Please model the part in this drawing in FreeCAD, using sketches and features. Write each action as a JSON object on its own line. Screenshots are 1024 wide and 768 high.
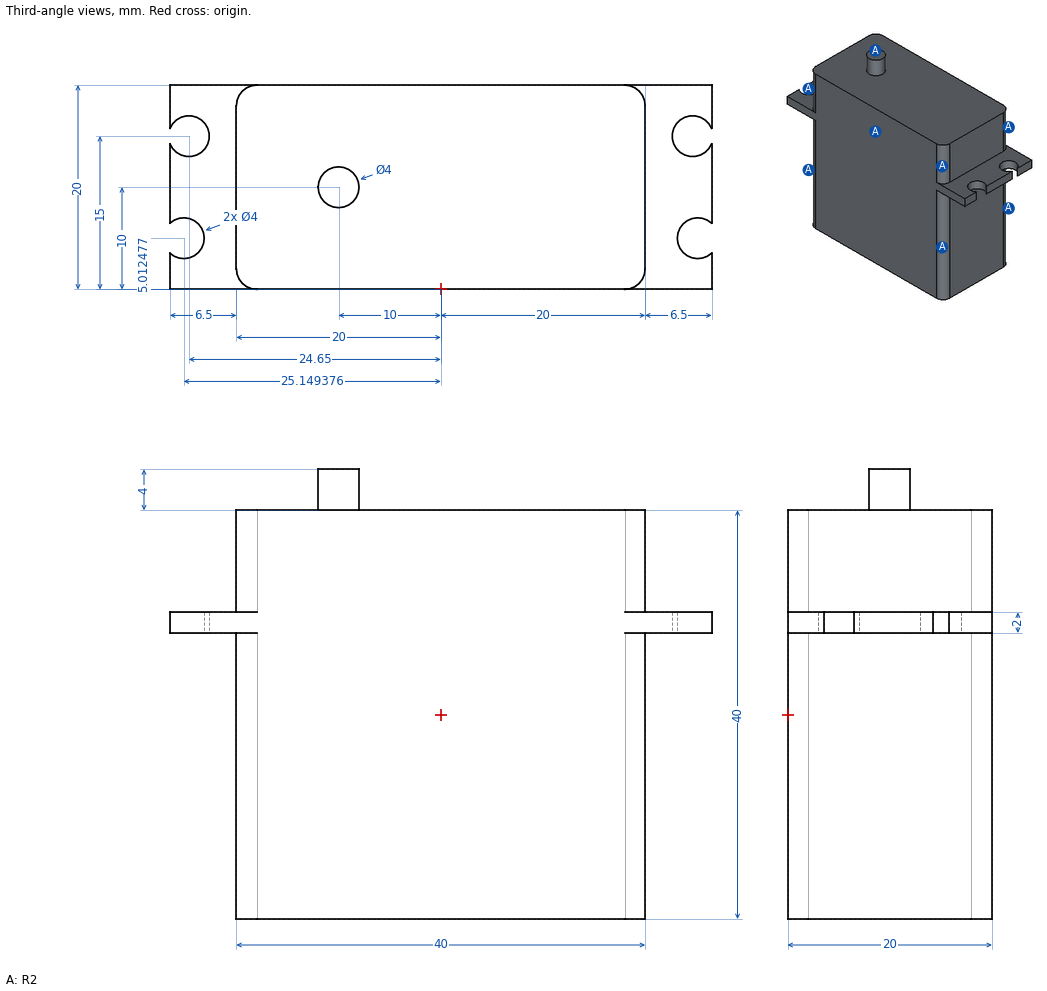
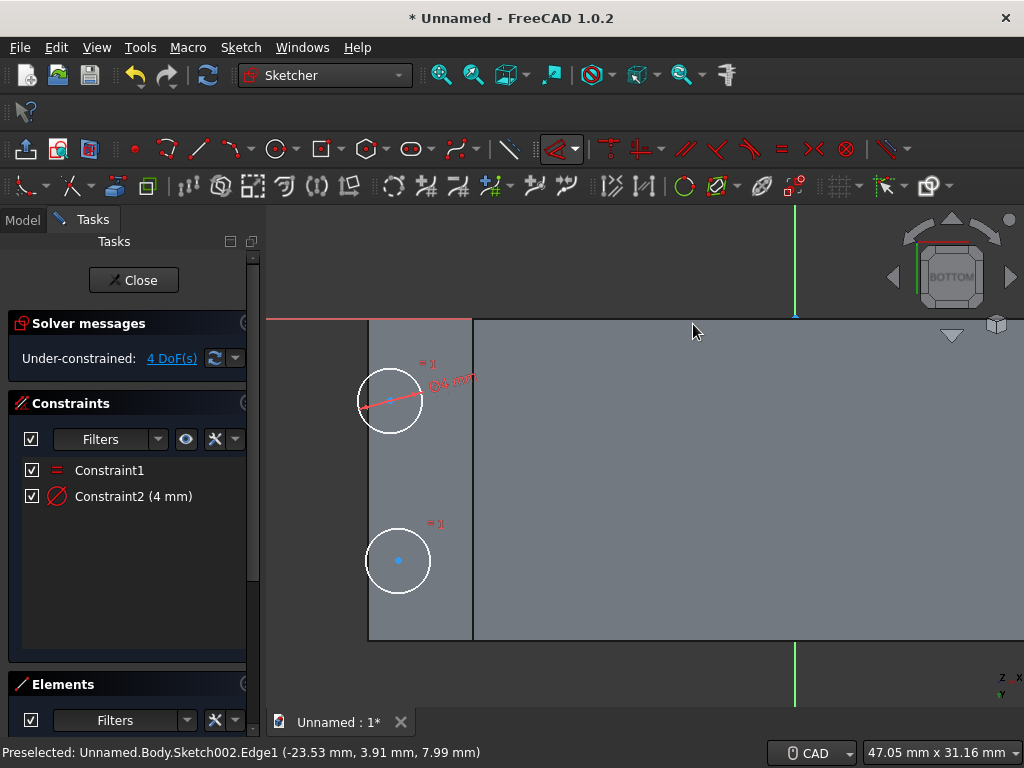
{"action": "left_click", "coordinate": [398, 561]}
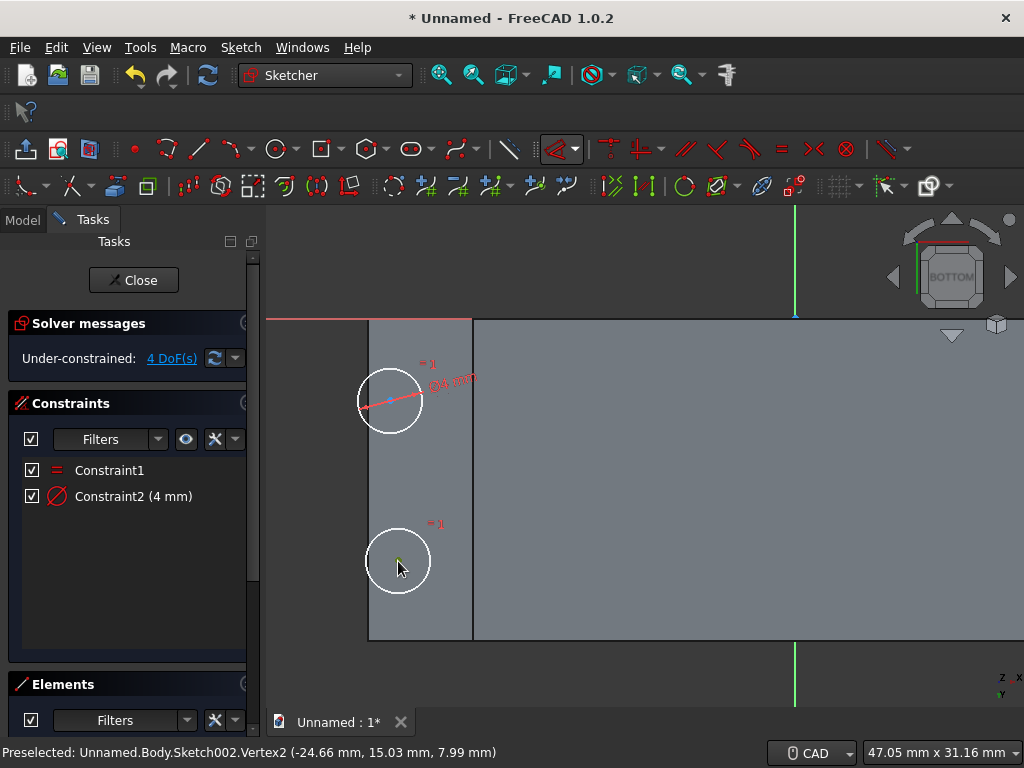
{"action": "left_click", "coordinate": [578, 150]}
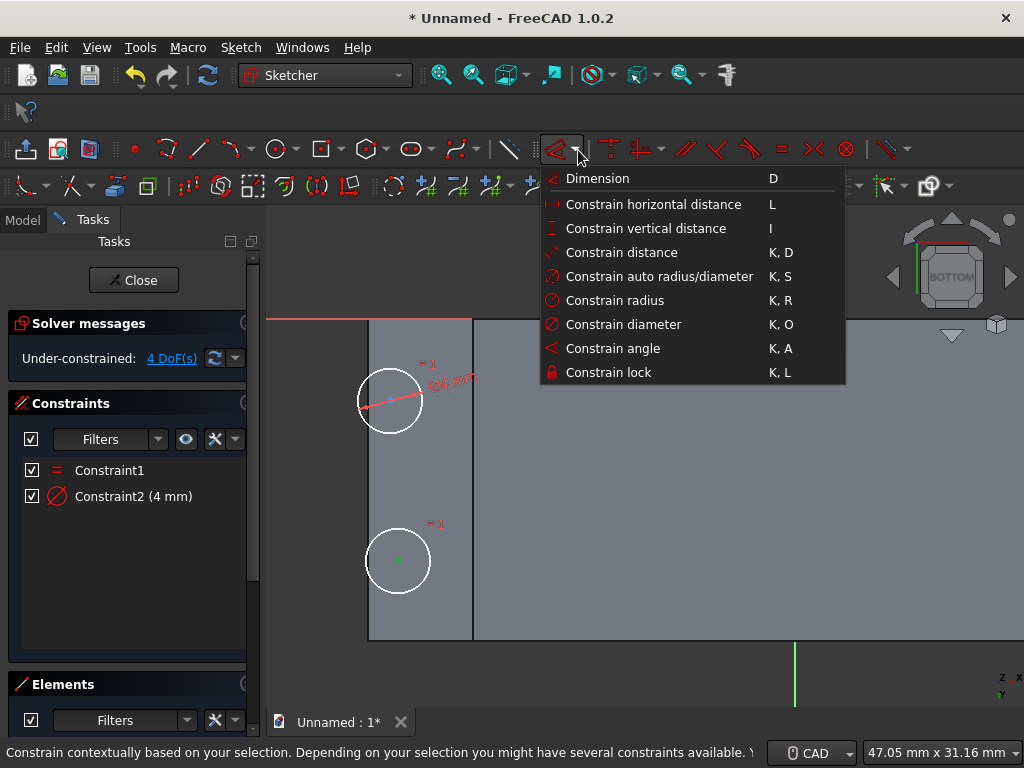
{"action": "left_click", "coordinate": [693, 228]}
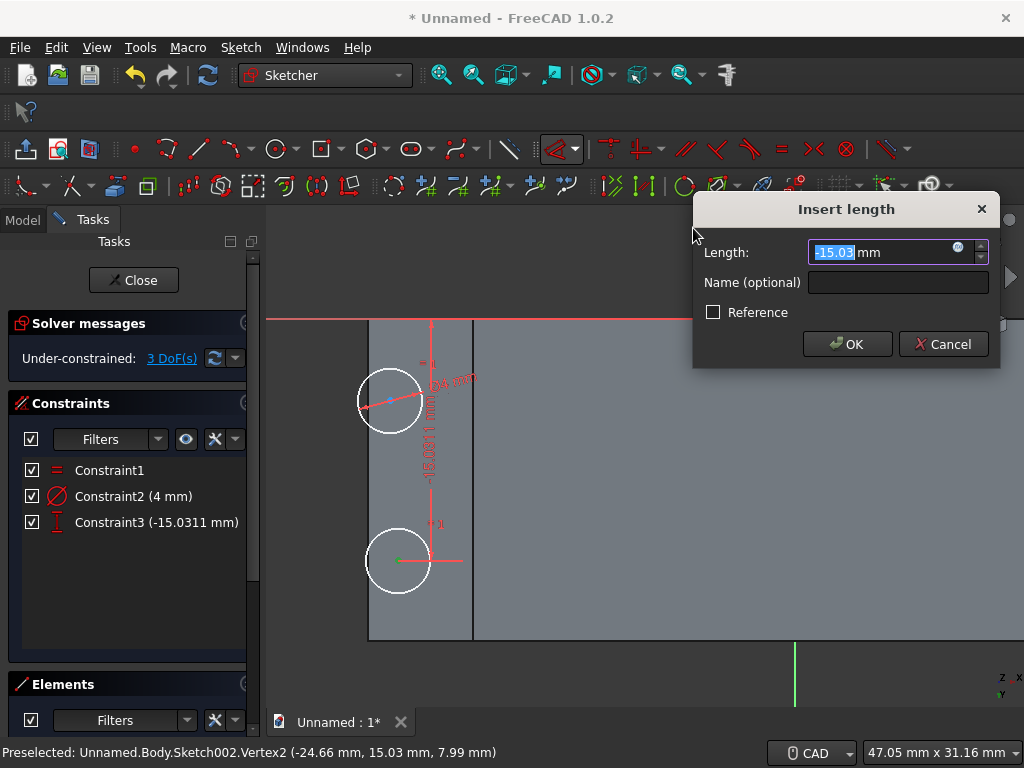
{"action": "type", "text": "-15"}
{"action": "key", "text": "Return"}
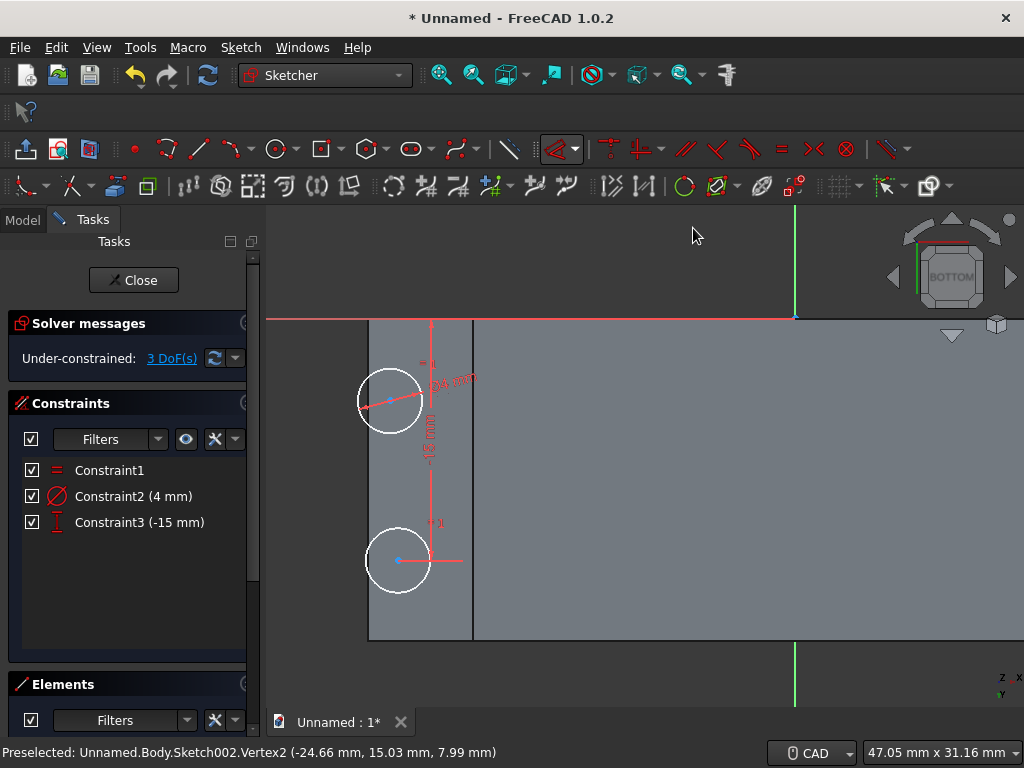
{"action": "left_click", "coordinate": [398, 560]}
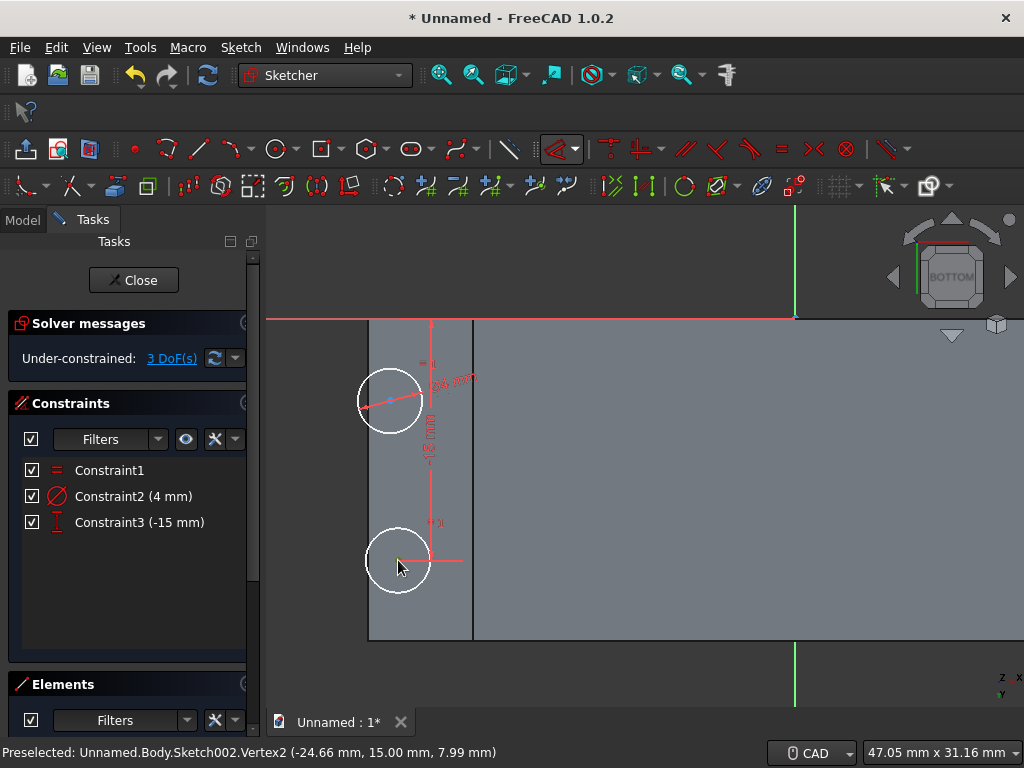
{"action": "key", "text": "l"}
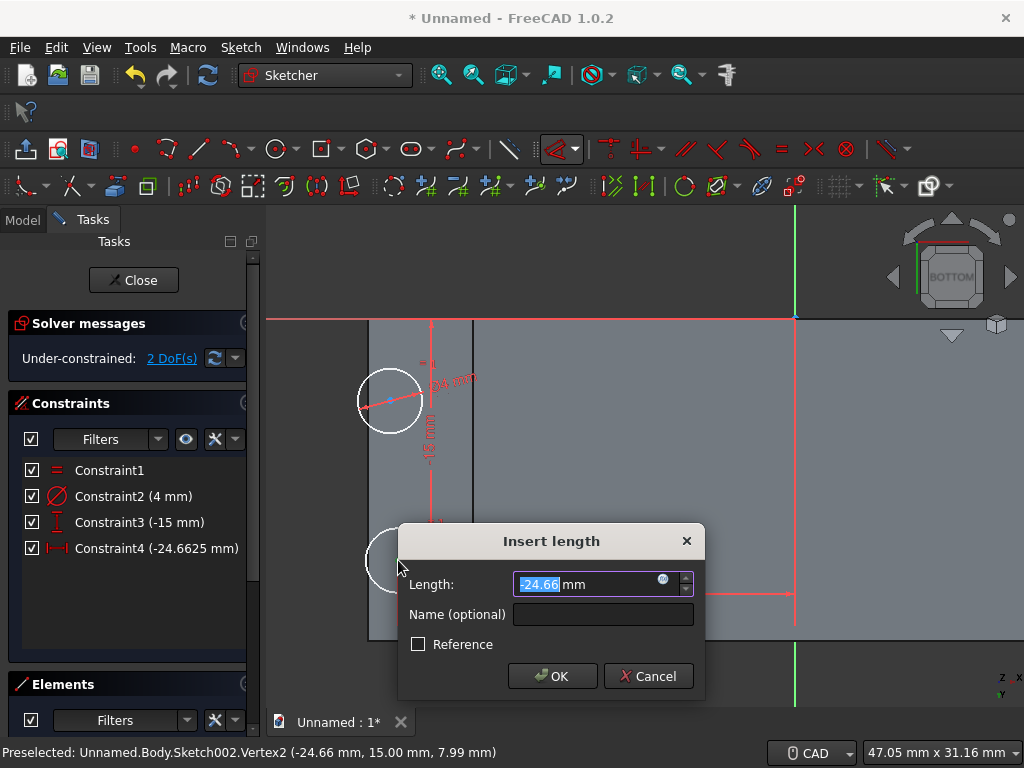
{"action": "type", "text": "-24.65"}
{"action": "key", "text": "Return"}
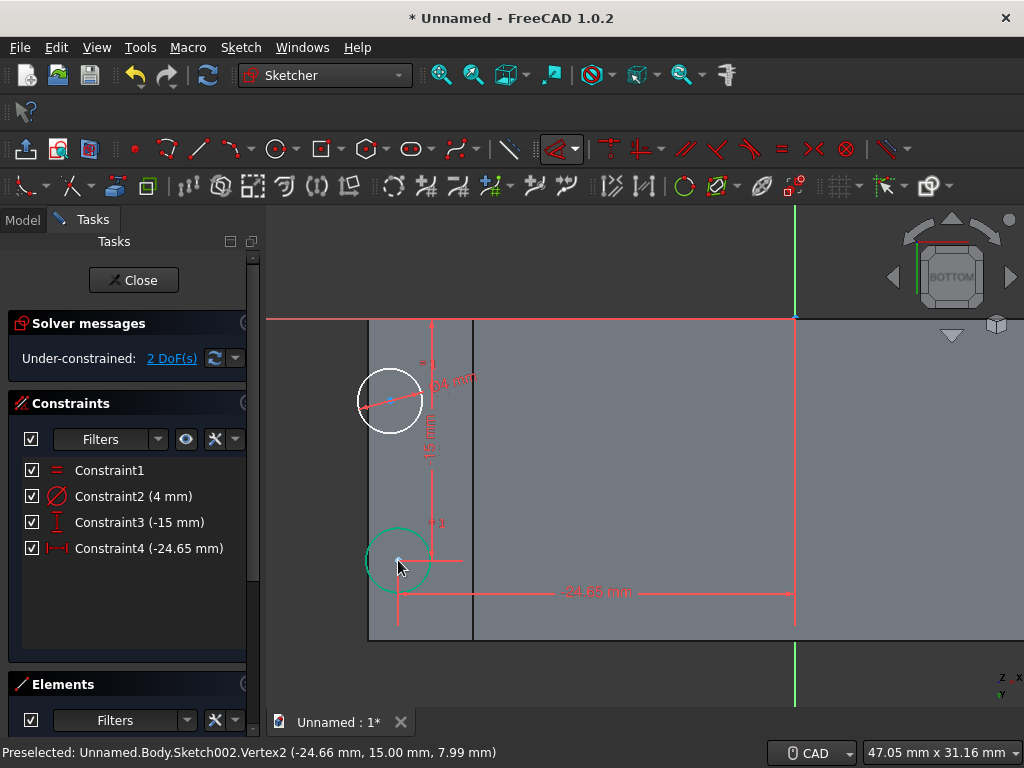
{"action": "left_click", "coordinate": [390, 401]}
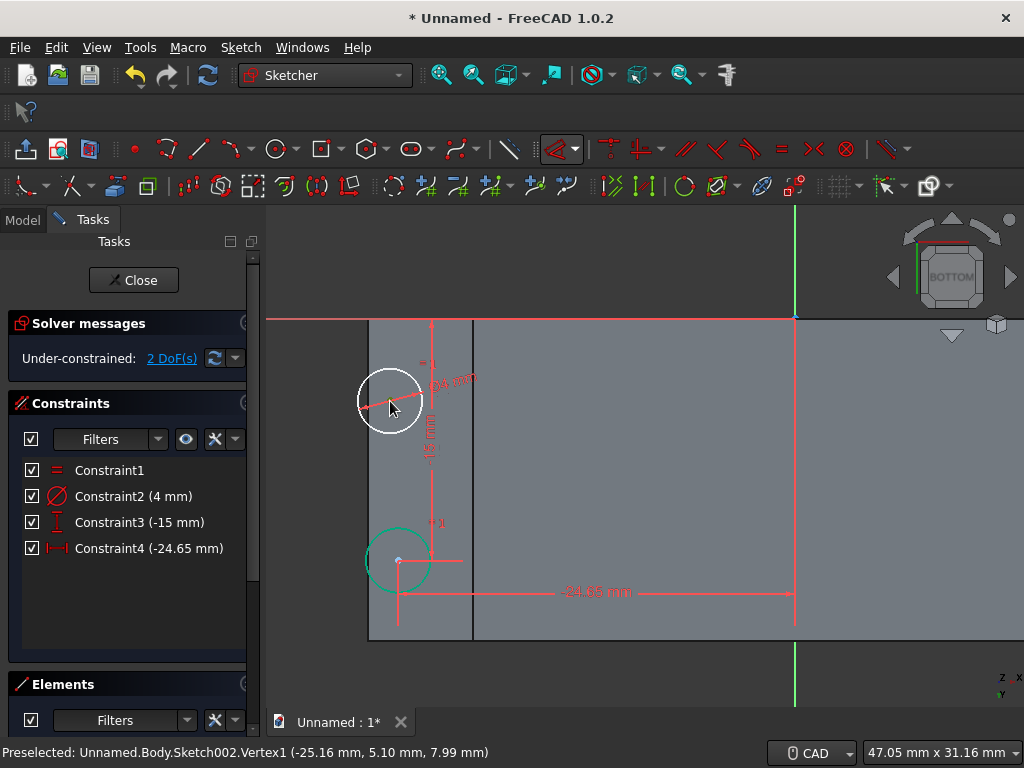
{"action": "key", "text": "i"}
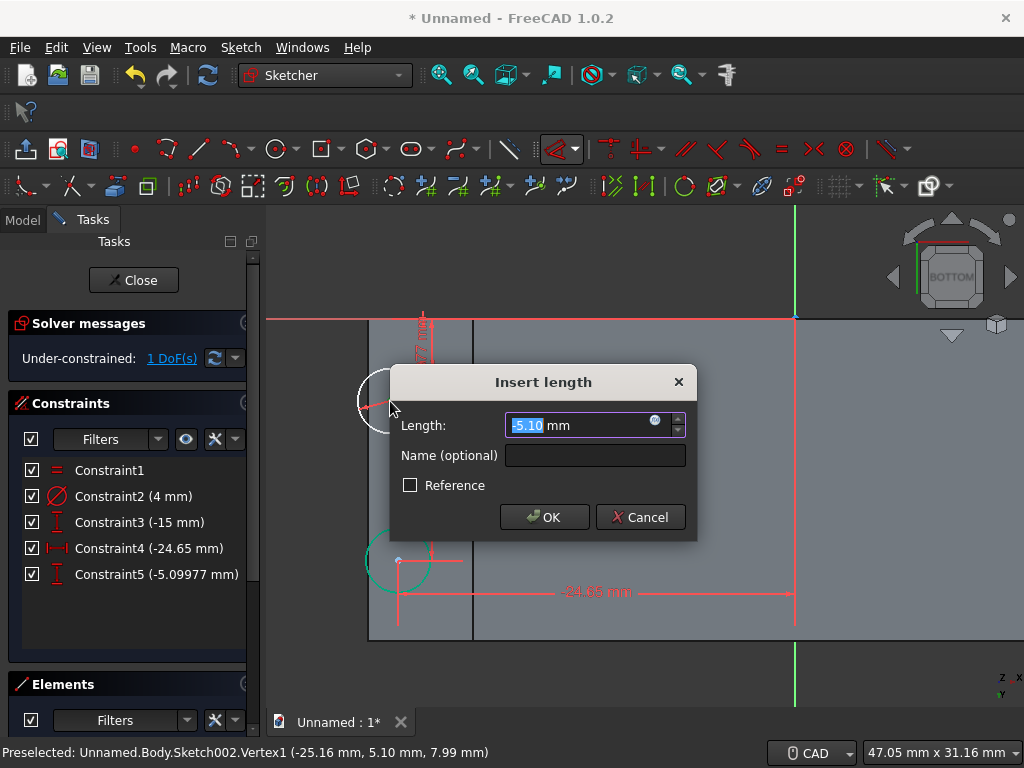
{"action": "type", "text": "-5.012477"}
{"action": "key", "text": "Return"}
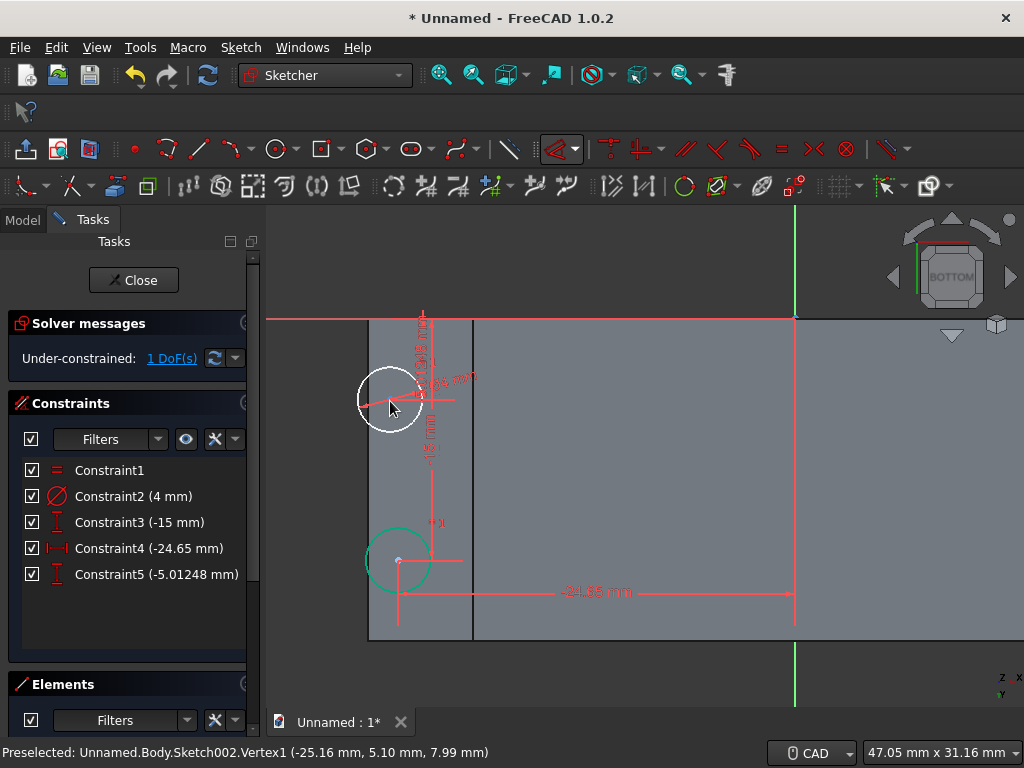
{"action": "left_click", "coordinate": [390, 400]}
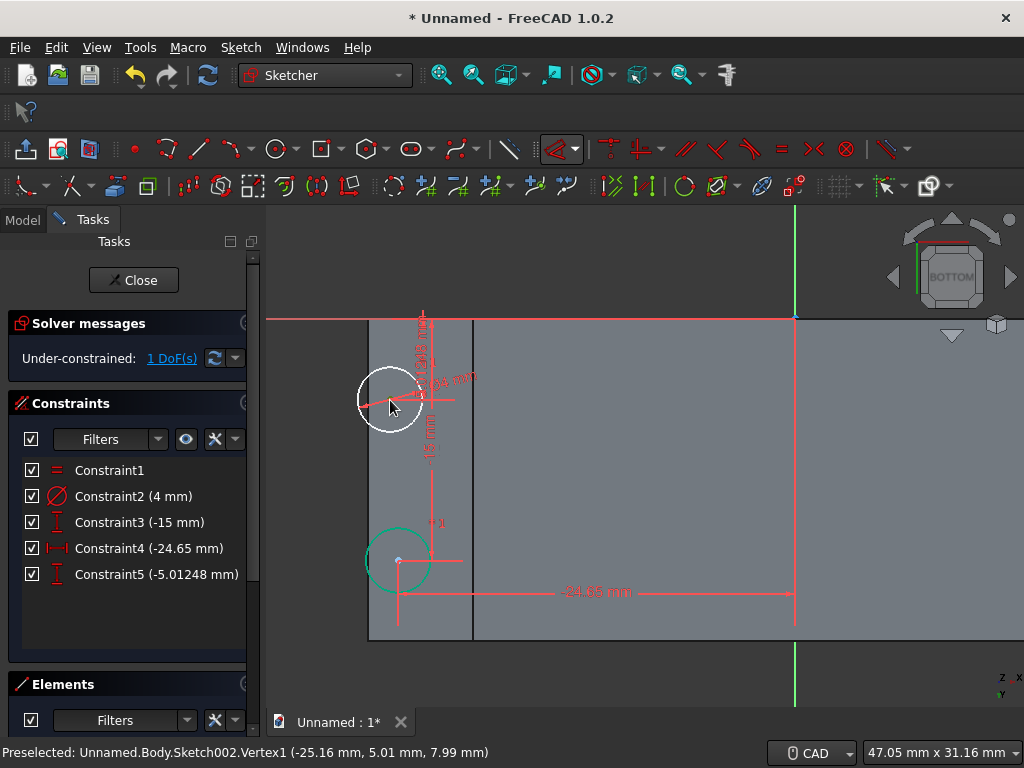
{"action": "left_click", "coordinate": [578, 150]}